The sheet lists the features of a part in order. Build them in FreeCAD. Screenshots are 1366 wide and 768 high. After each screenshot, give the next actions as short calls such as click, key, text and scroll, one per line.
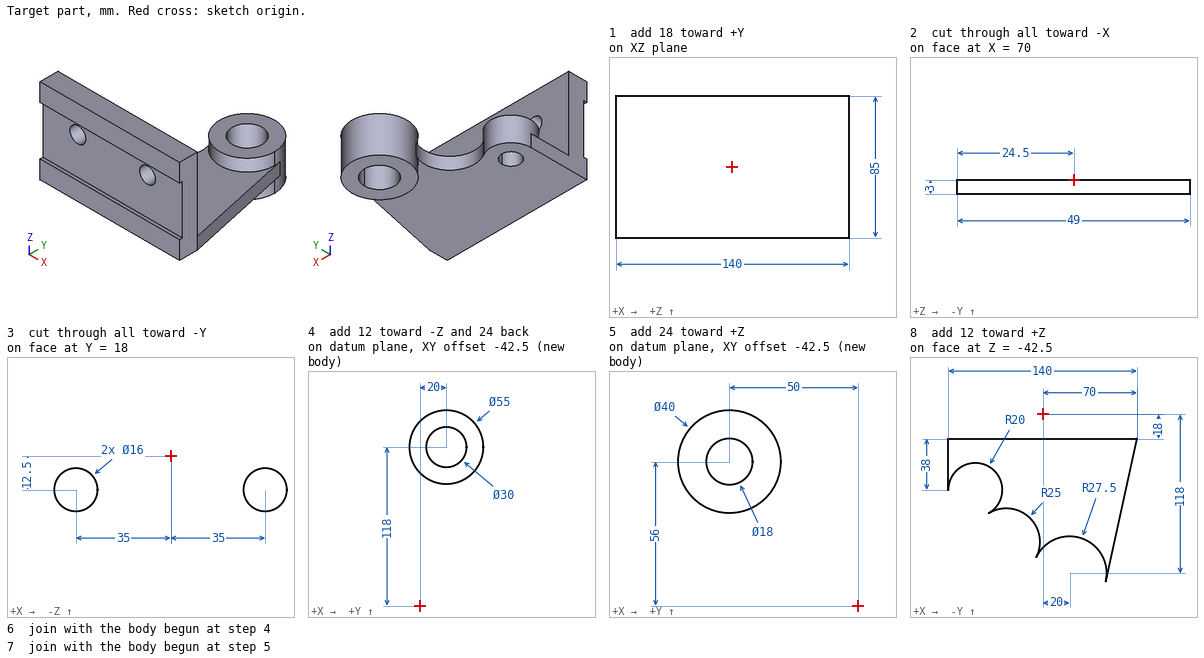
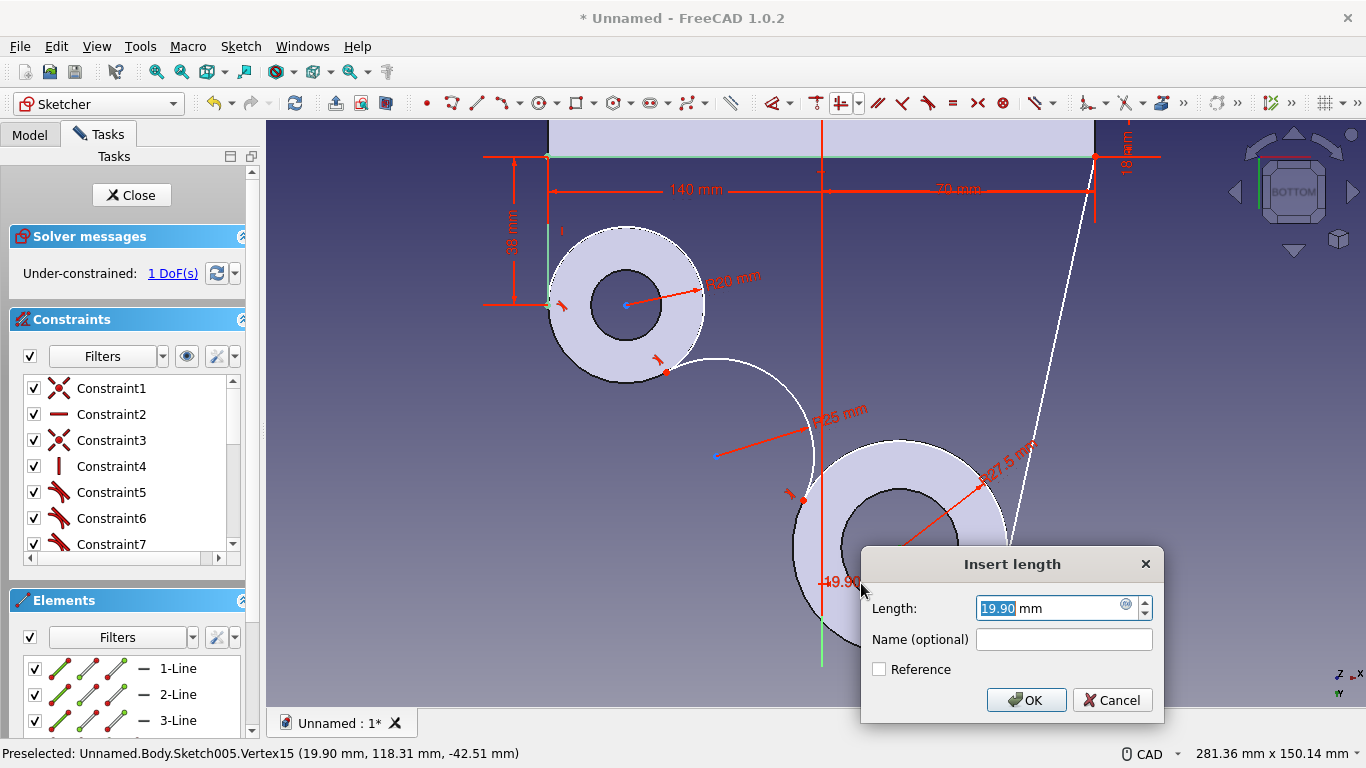
text(20)
key(Return)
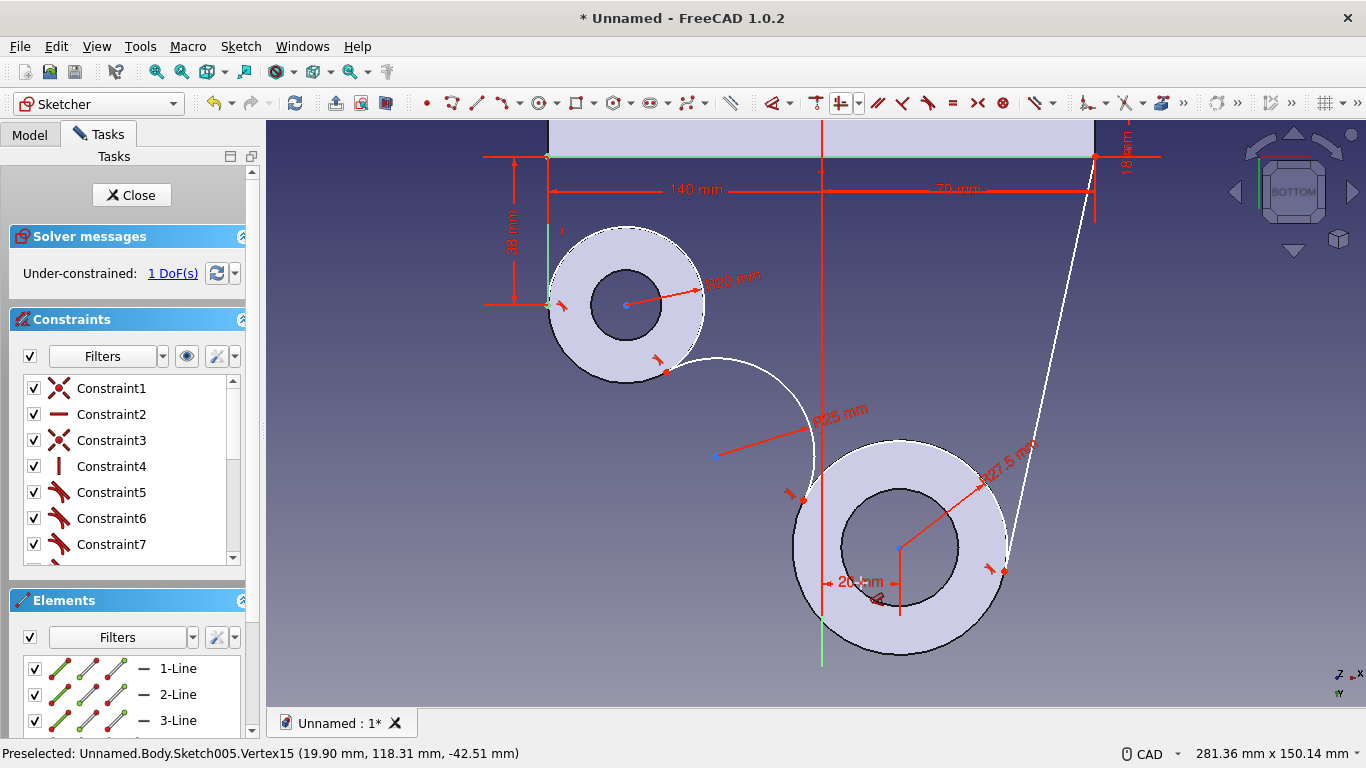
click(900, 549)
click(934, 348)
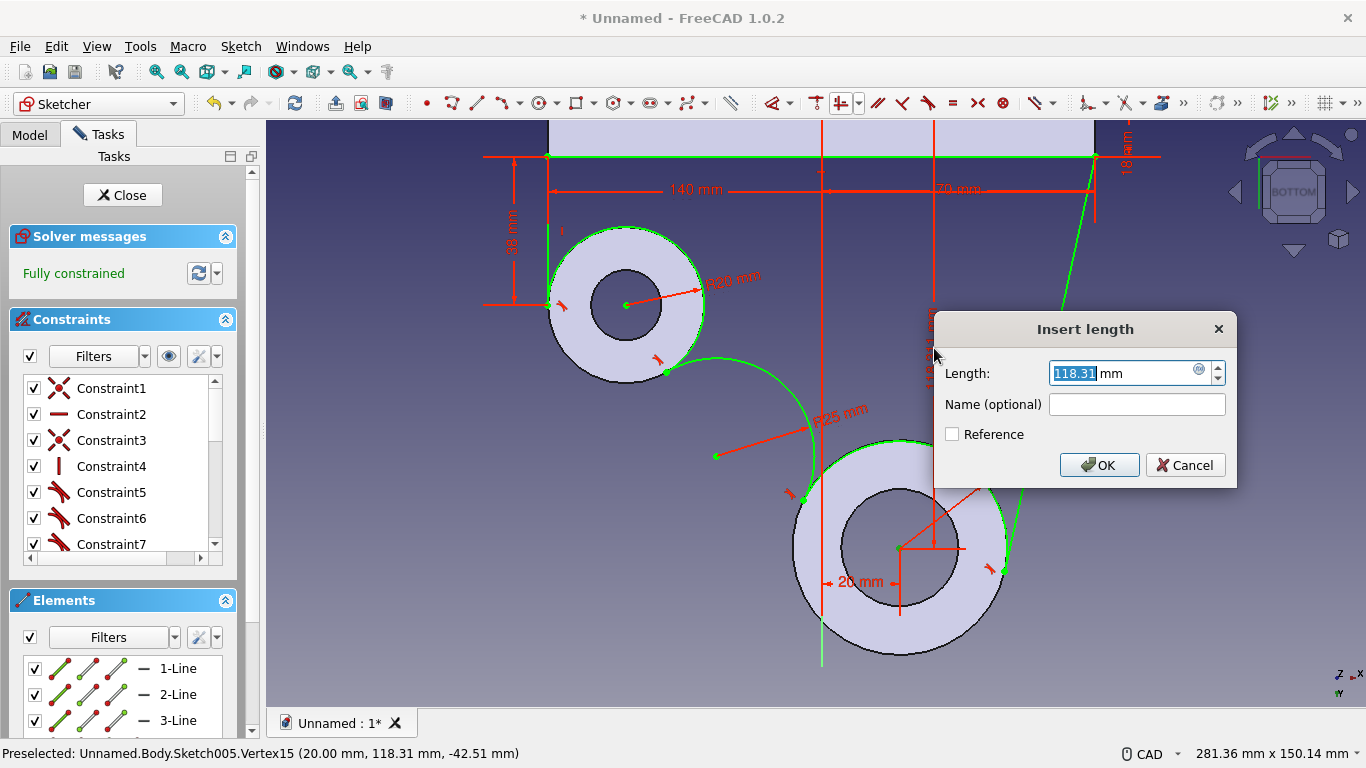
text(118)
key(Return)
key(Escape)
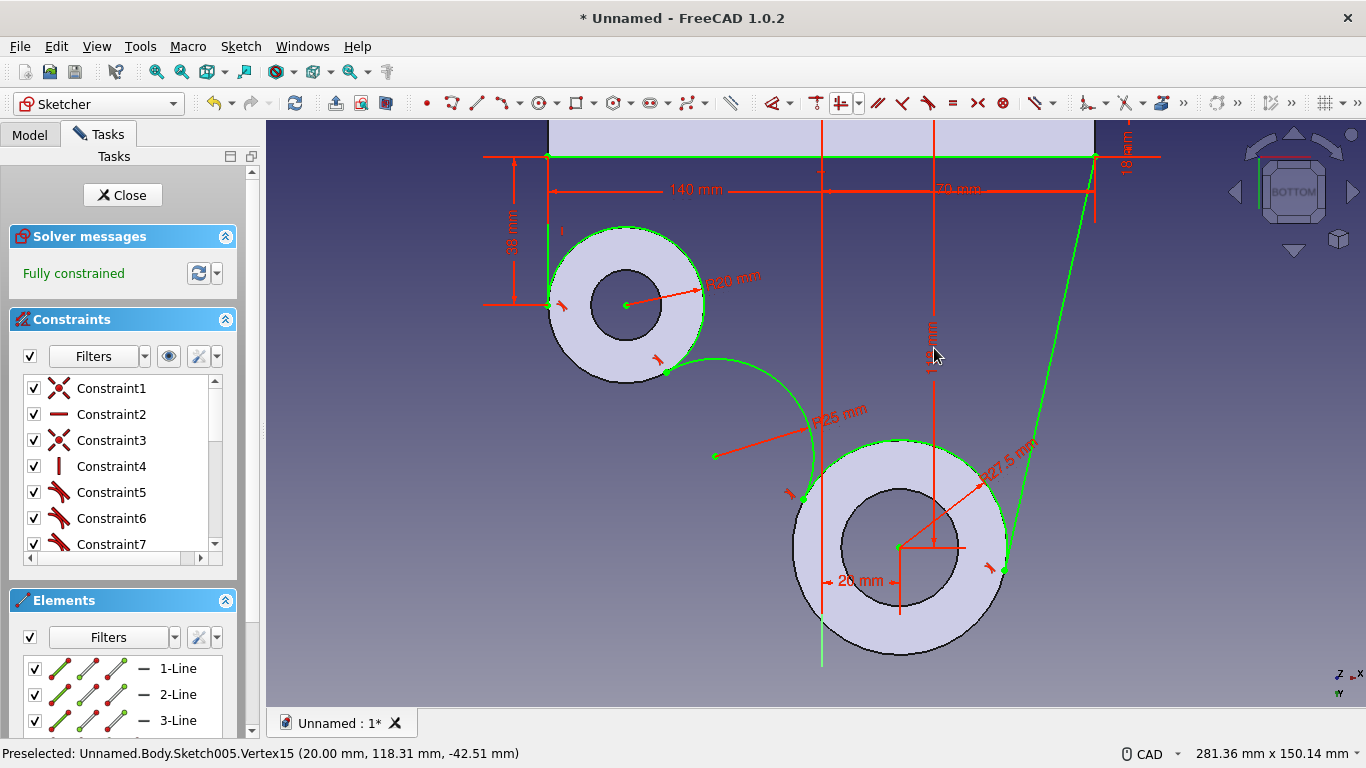
click(123, 195)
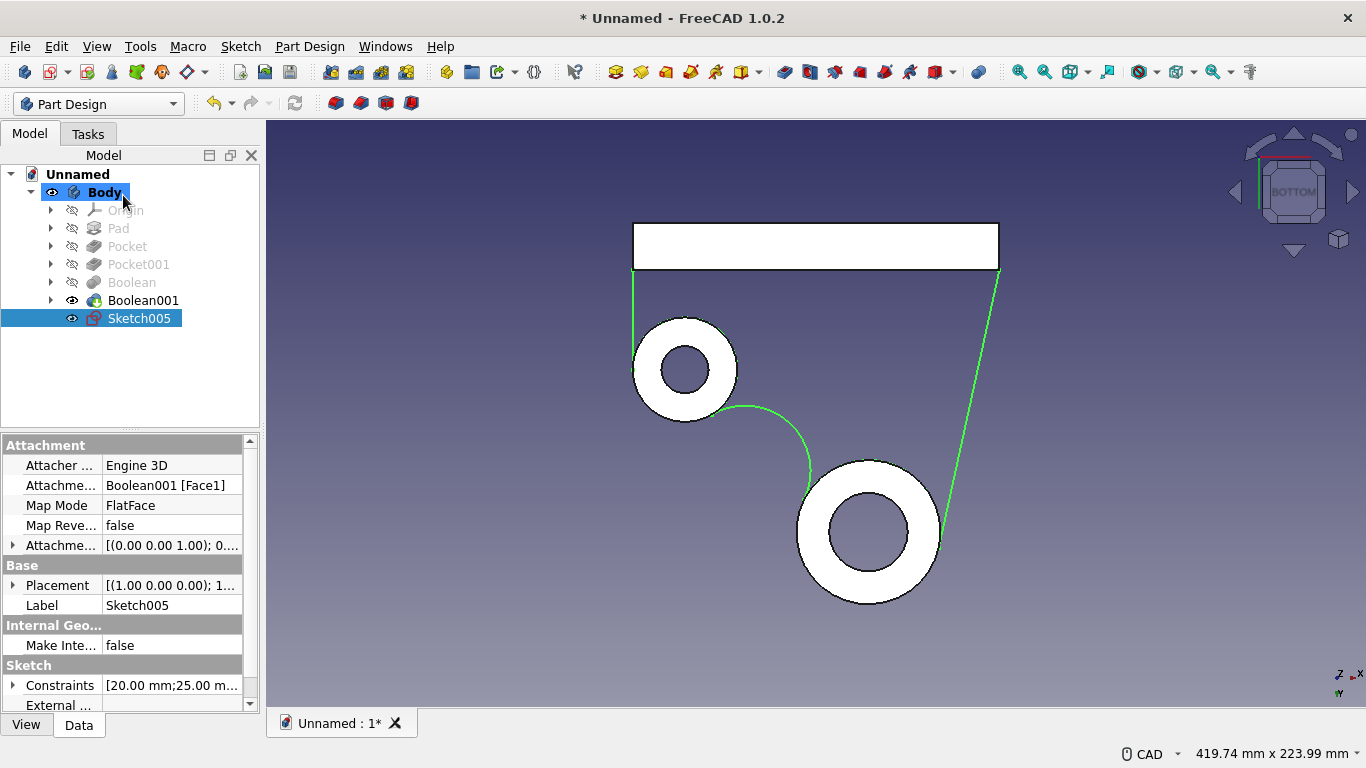
click(616, 72)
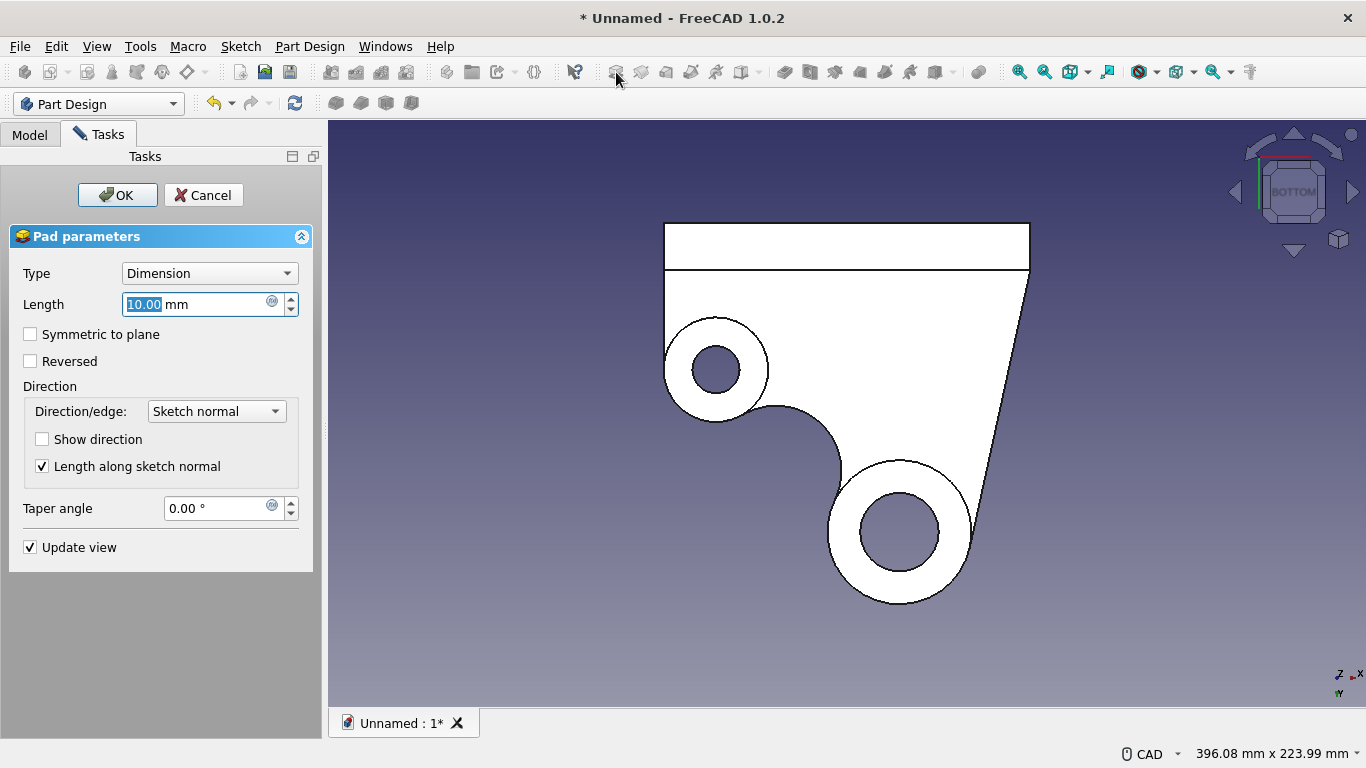
text(12)
key(Tab)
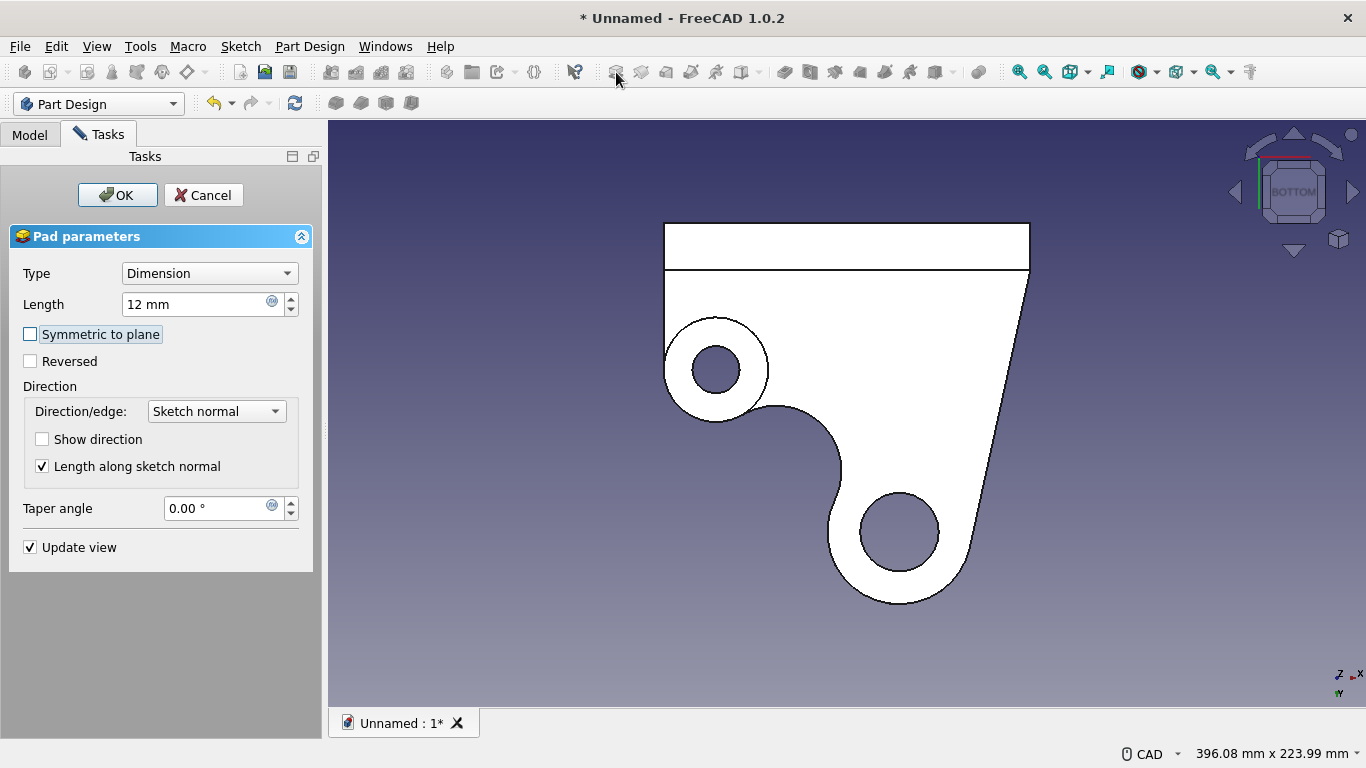
click(31, 361)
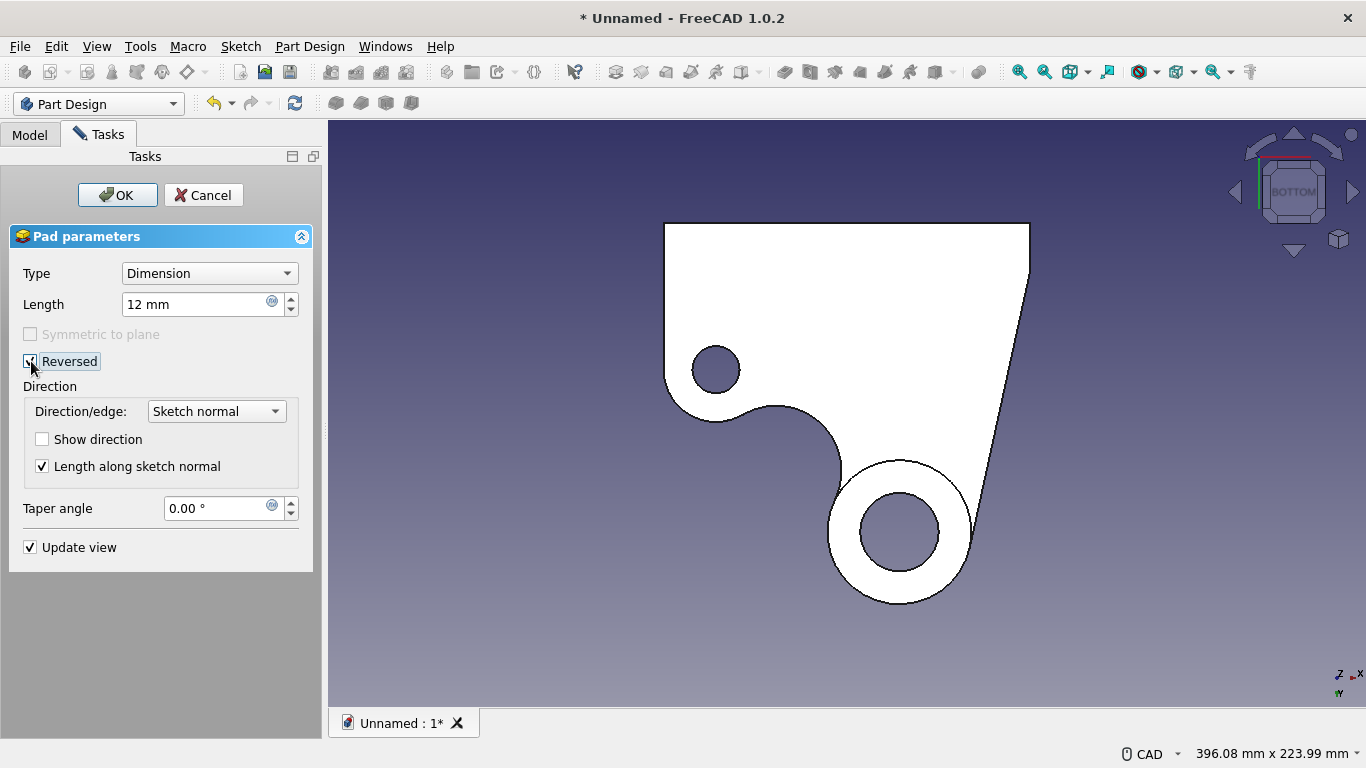
click(118, 195)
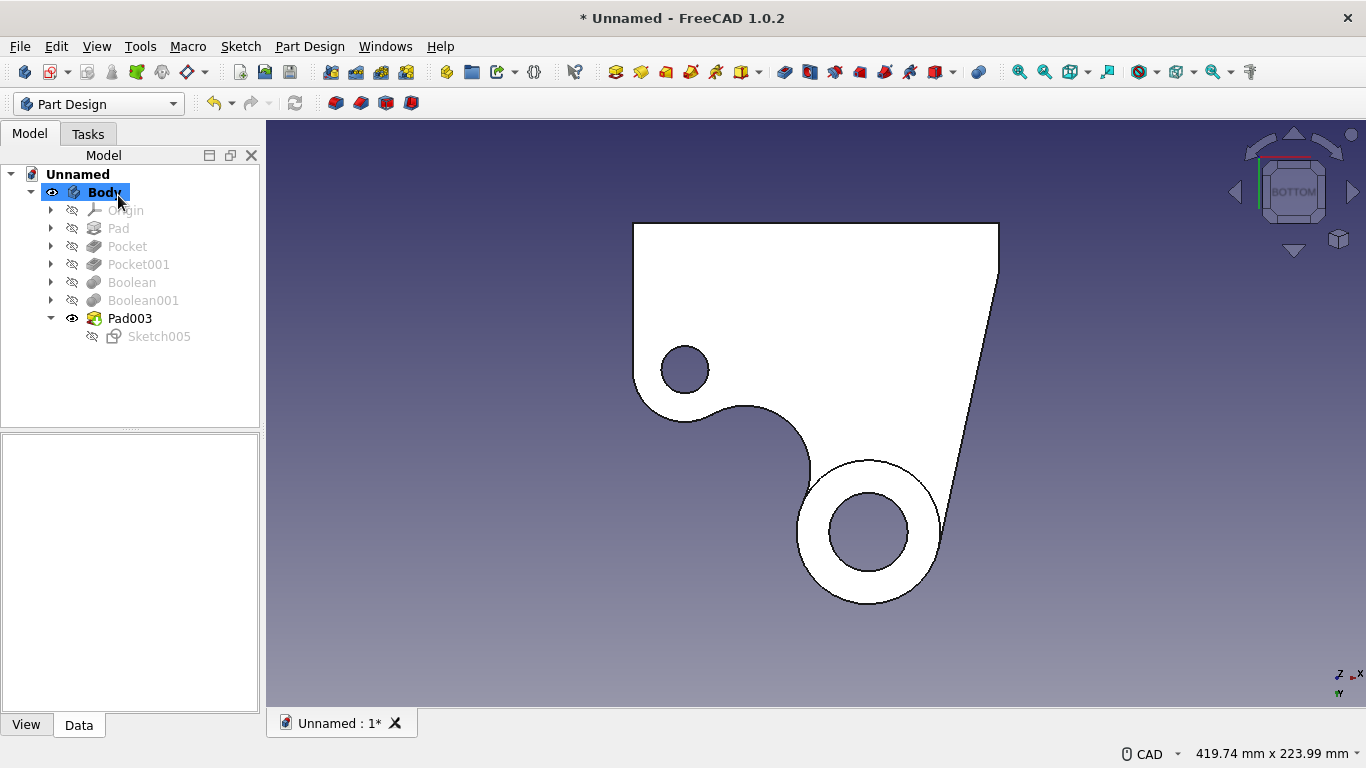
key(0)